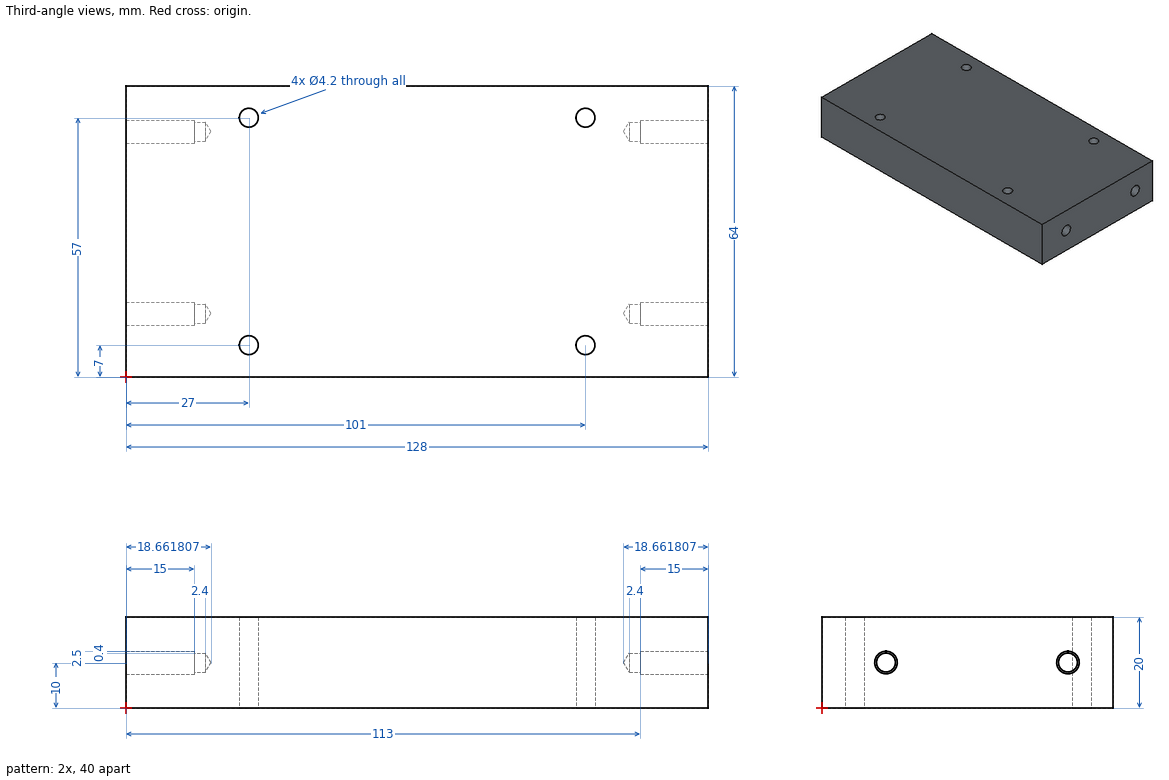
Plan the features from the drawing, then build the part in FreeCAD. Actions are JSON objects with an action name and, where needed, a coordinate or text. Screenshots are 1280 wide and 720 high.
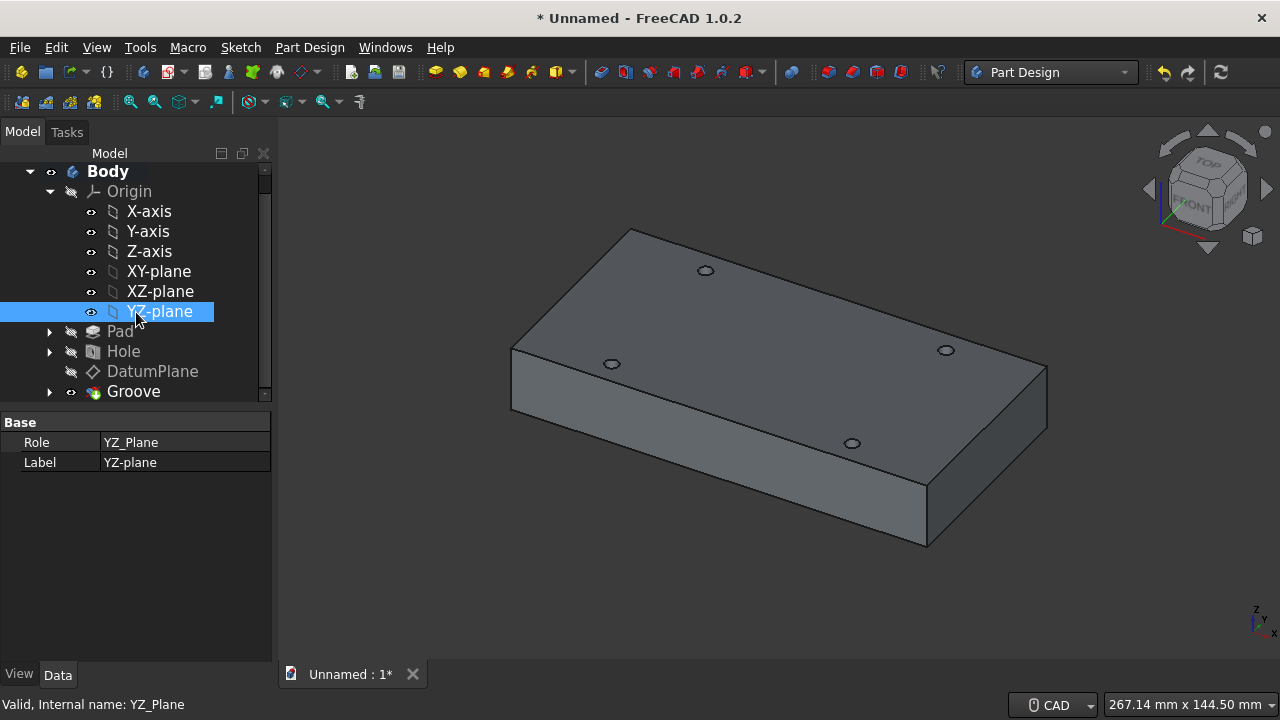
{"action": "left_click", "coordinate": [302, 72]}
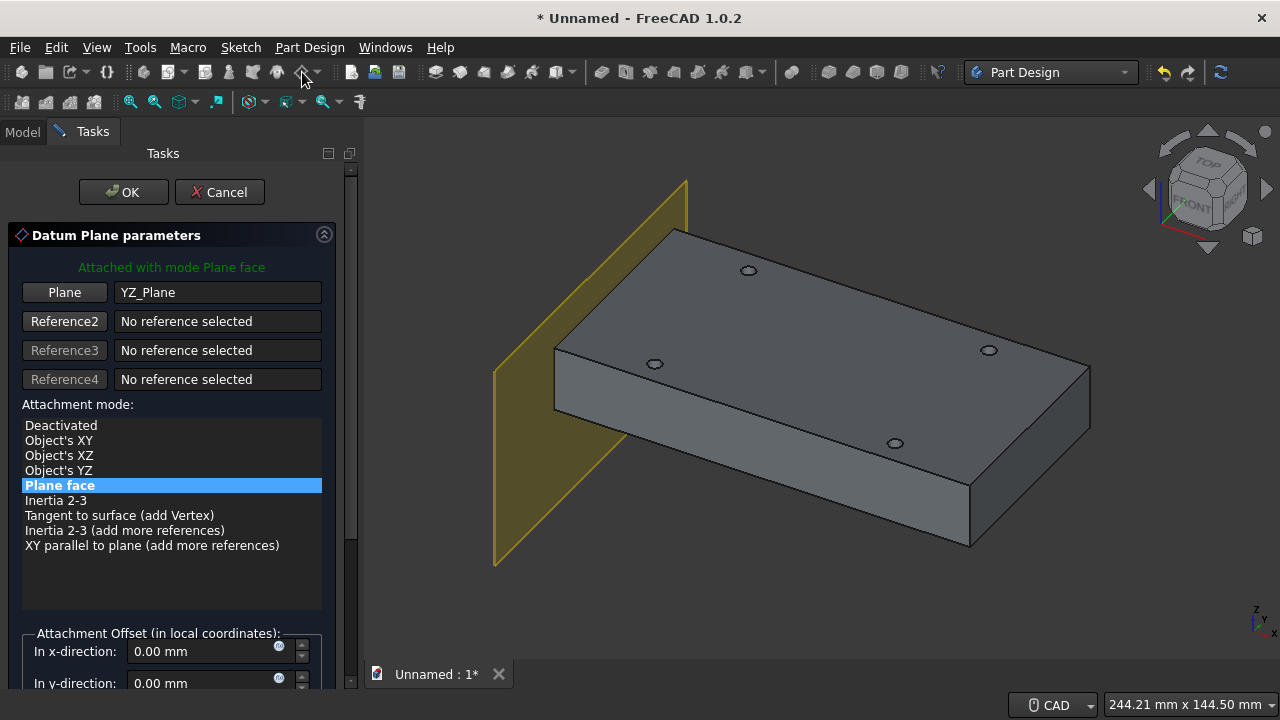
{"action": "scroll", "coordinate": [351, 426], "scroll_direction": "down", "scroll_amount": 2}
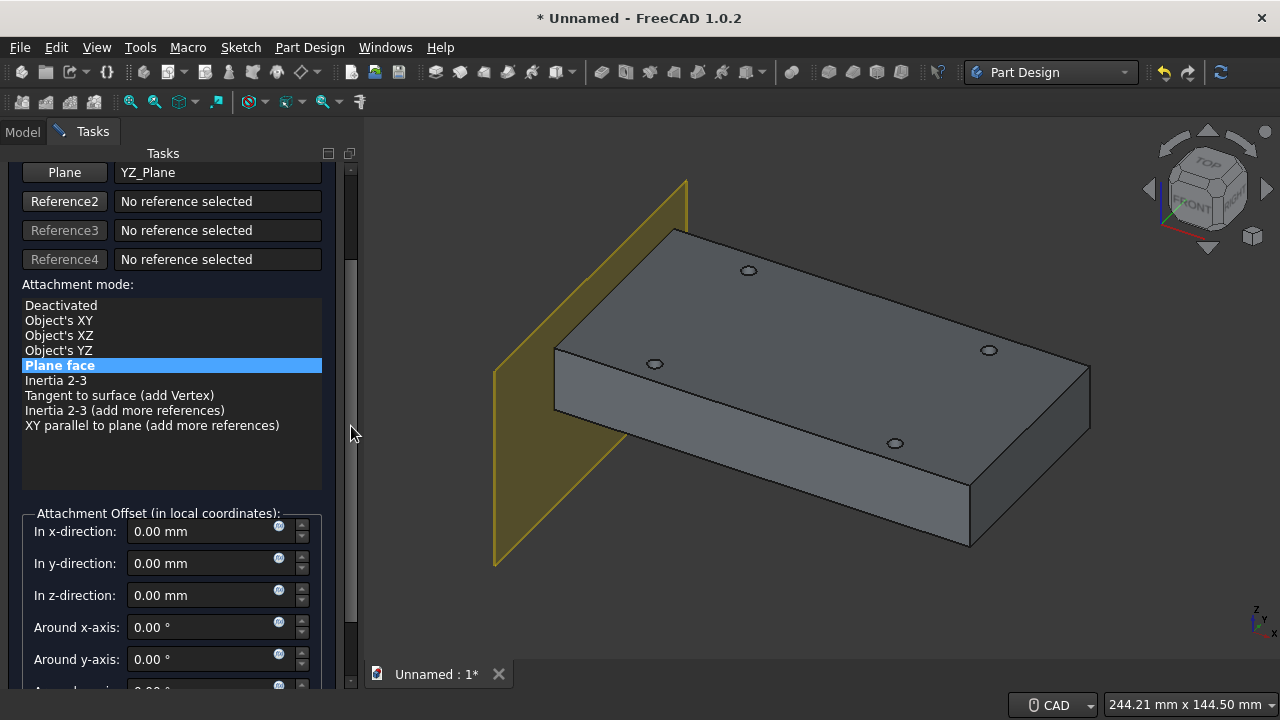
{"action": "triple_click", "coordinate": [210, 595]}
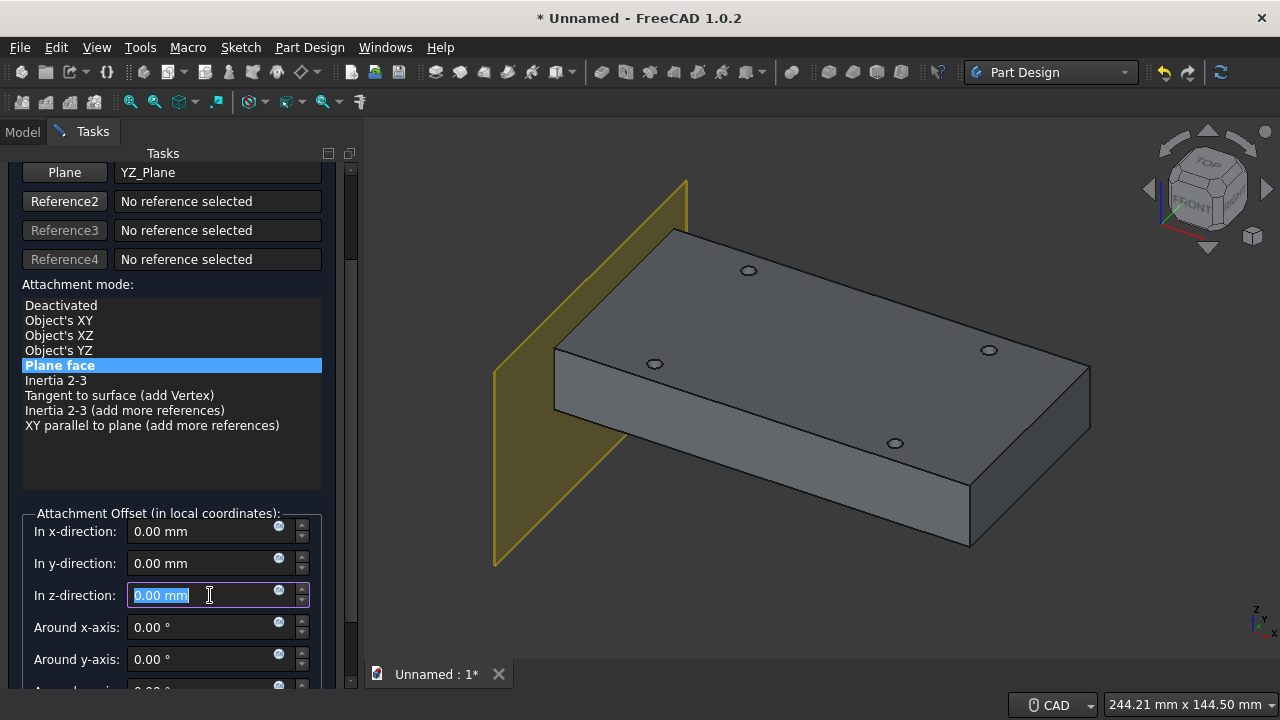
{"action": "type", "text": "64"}
{"action": "key", "text": "Tab"}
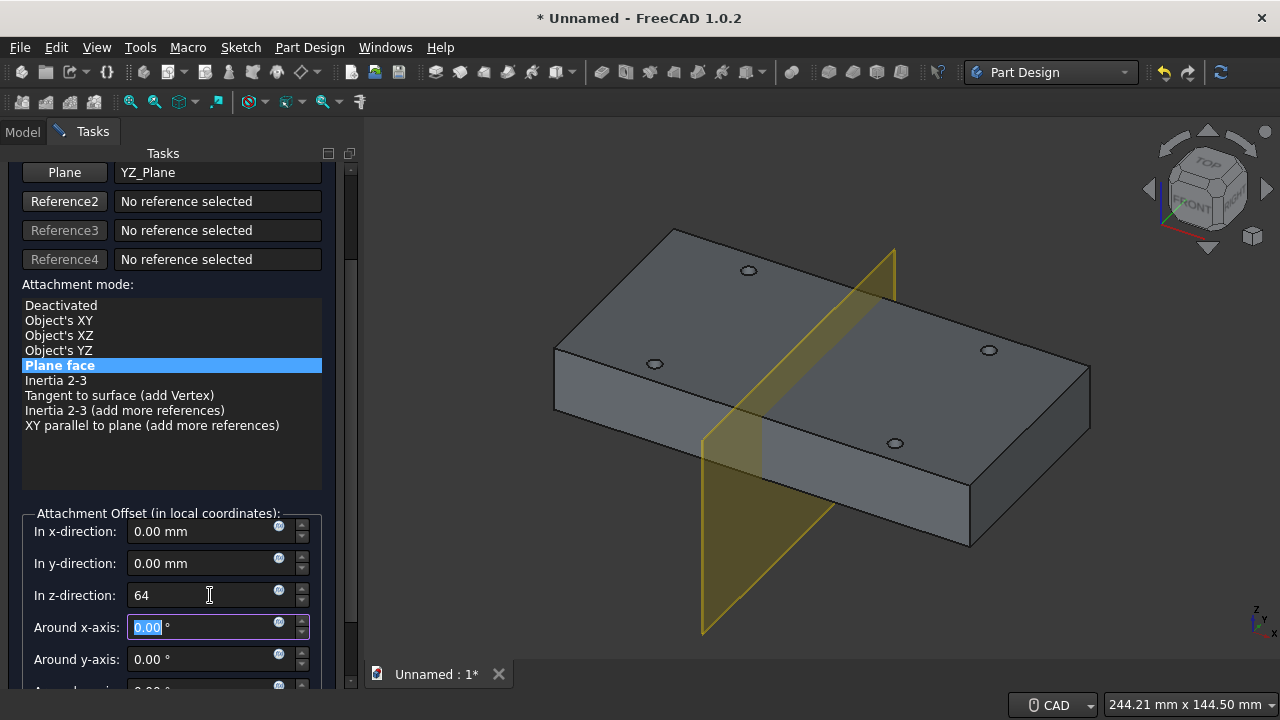
{"action": "scroll", "coordinate": [351, 426], "scroll_direction": "up", "scroll_amount": 3}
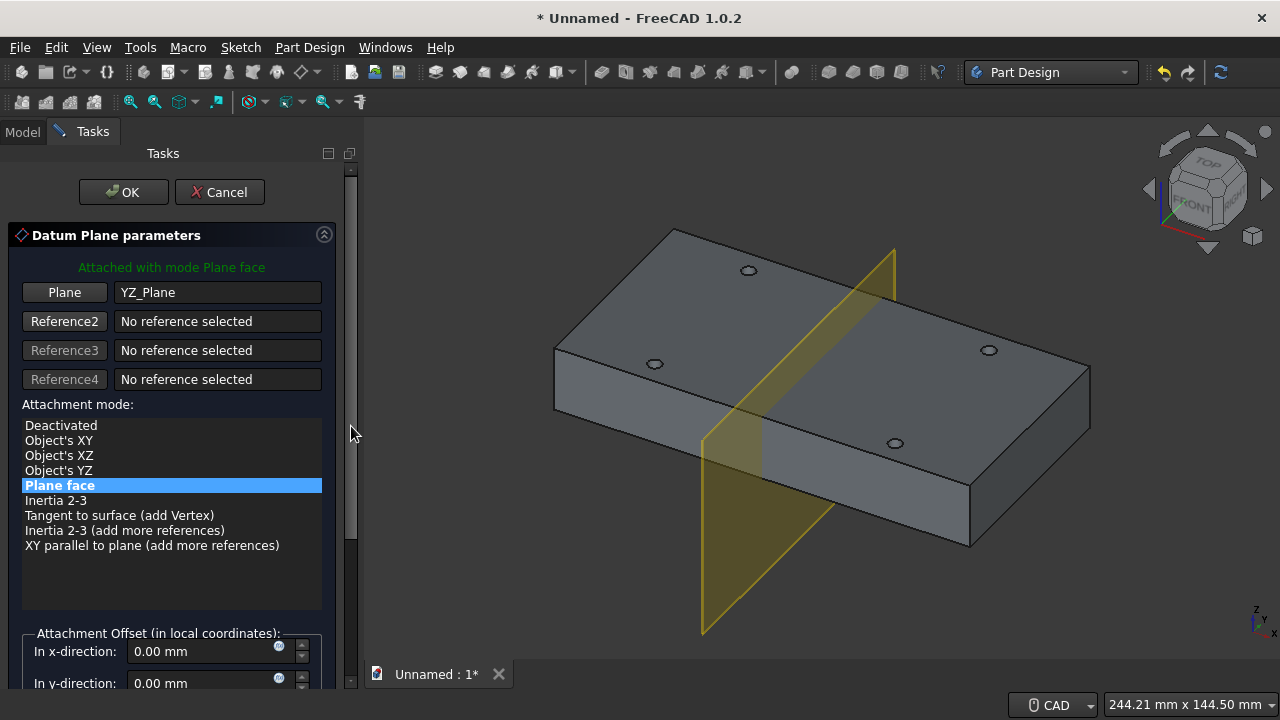
{"action": "left_click", "coordinate": [124, 192]}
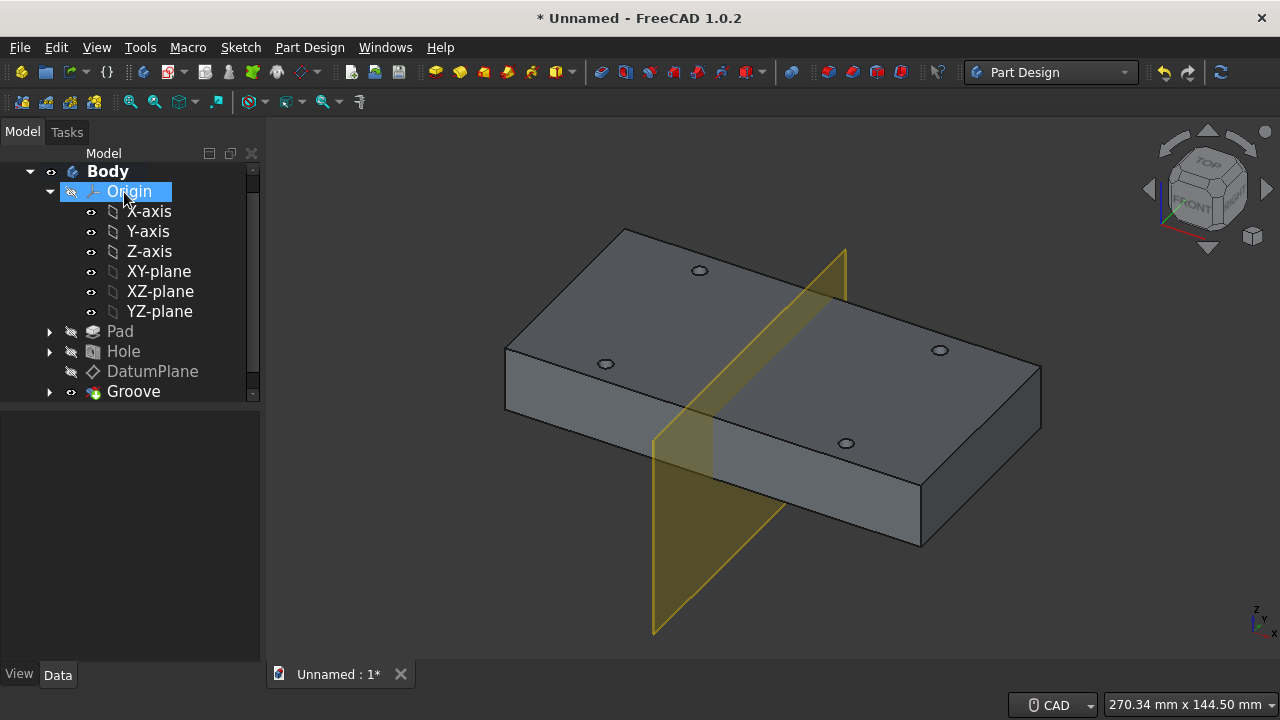
{"action": "left_click", "coordinate": [116, 392]}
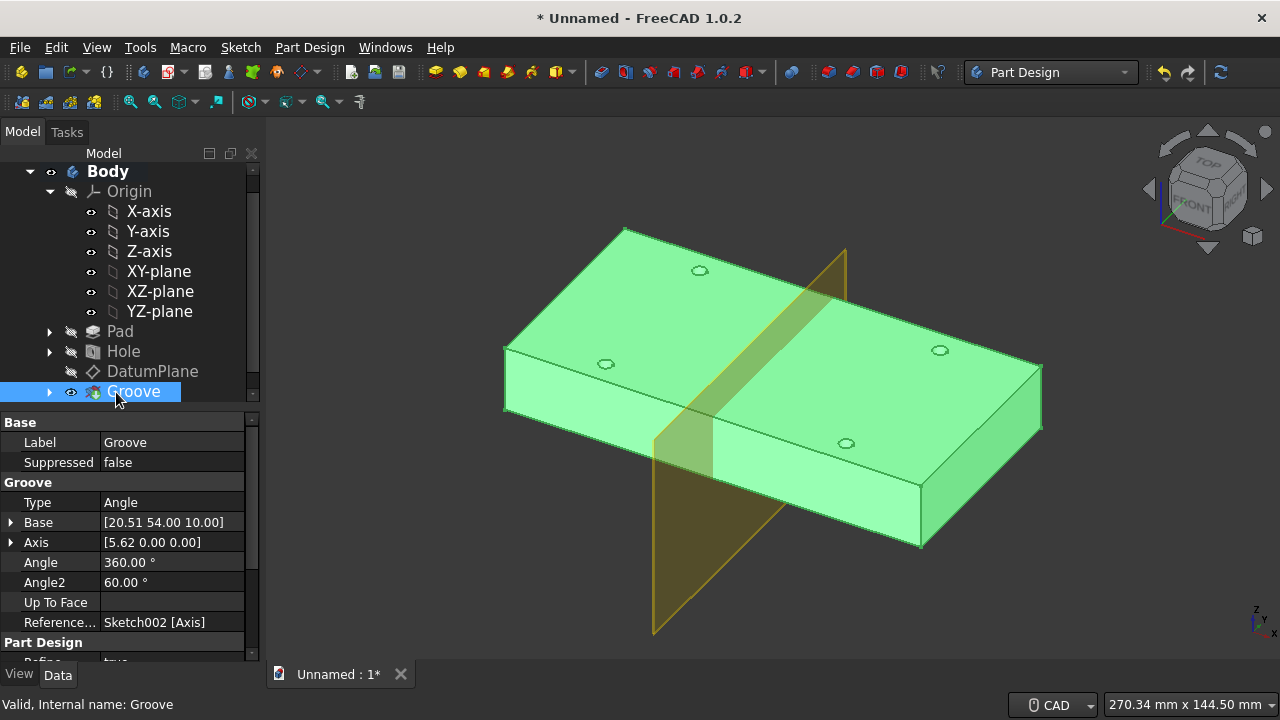
{"action": "left_click", "coordinate": [22, 102]}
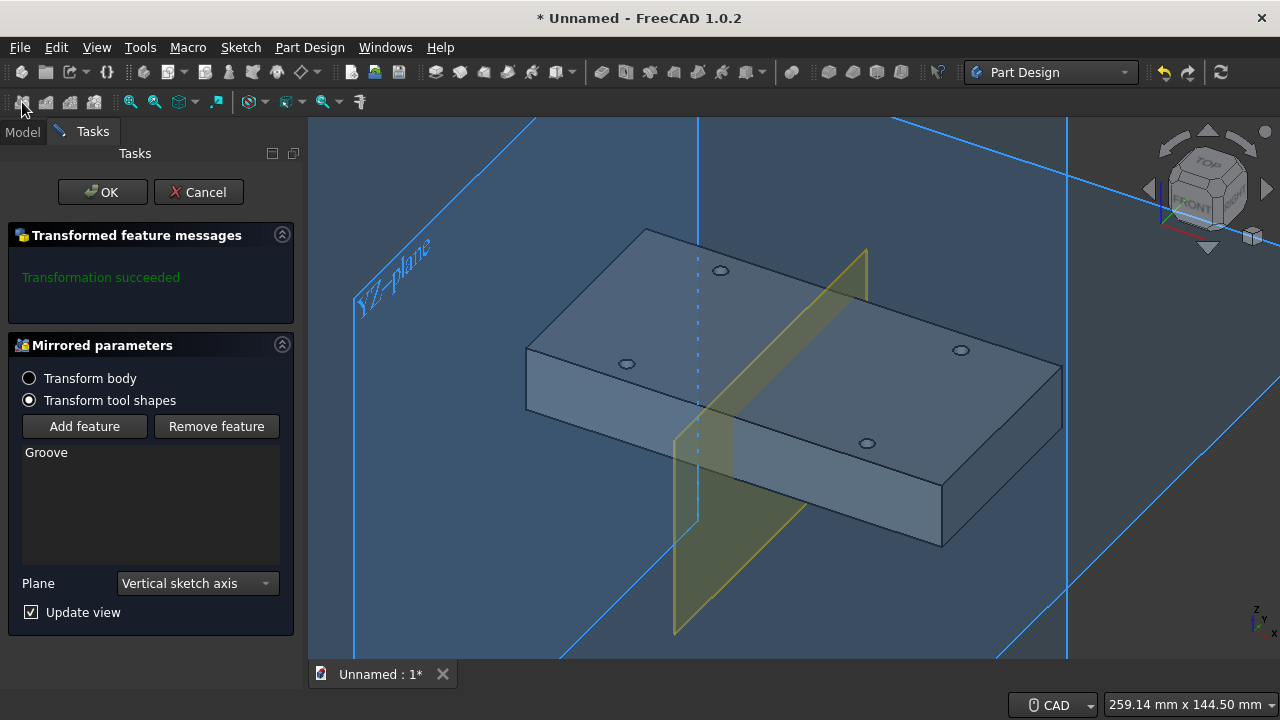
{"action": "left_click", "coordinate": [198, 584]}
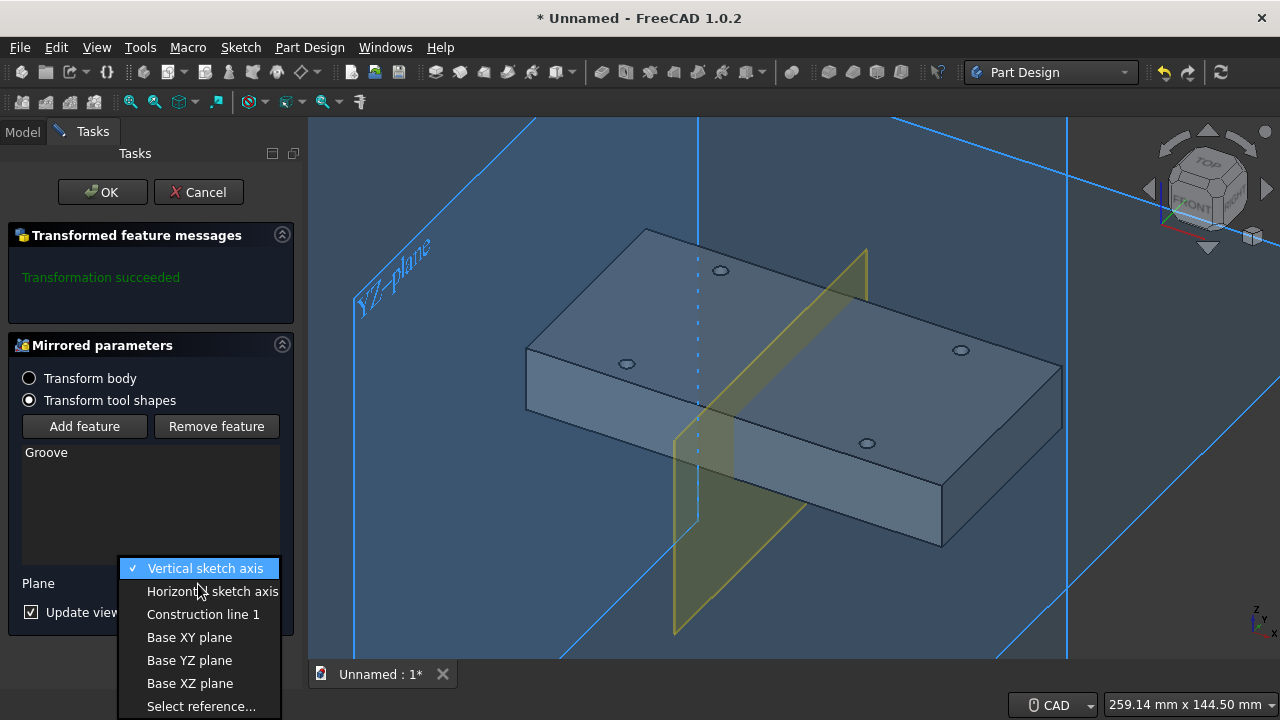
{"action": "left_click", "coordinate": [198, 706]}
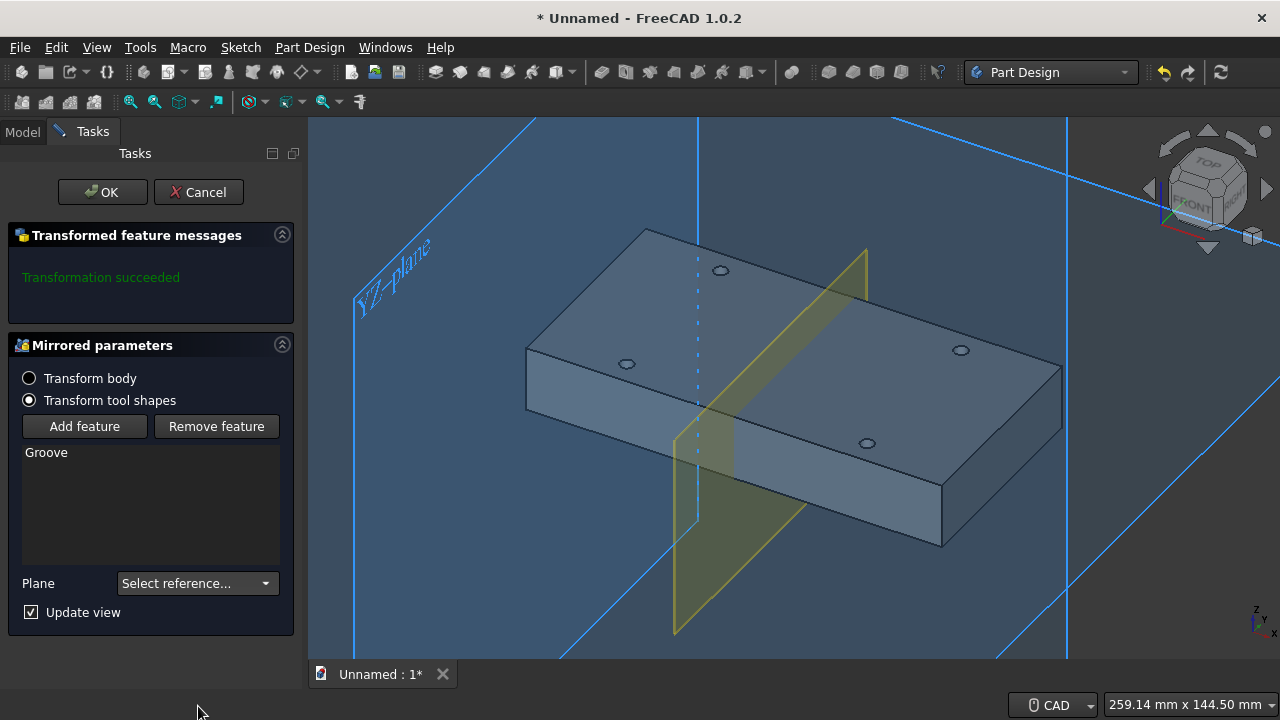
{"action": "left_click", "coordinate": [23, 131]}